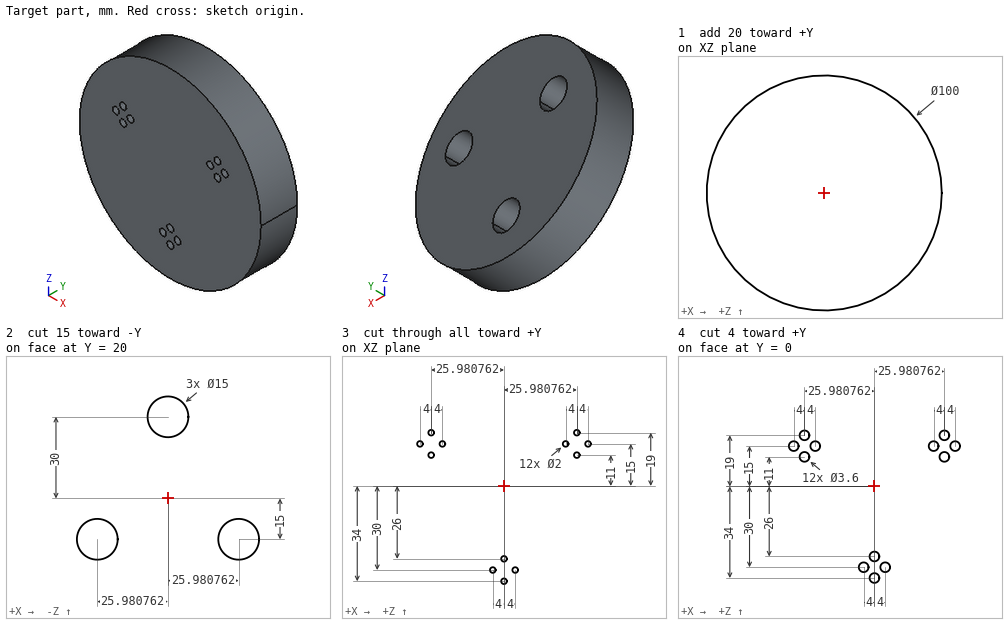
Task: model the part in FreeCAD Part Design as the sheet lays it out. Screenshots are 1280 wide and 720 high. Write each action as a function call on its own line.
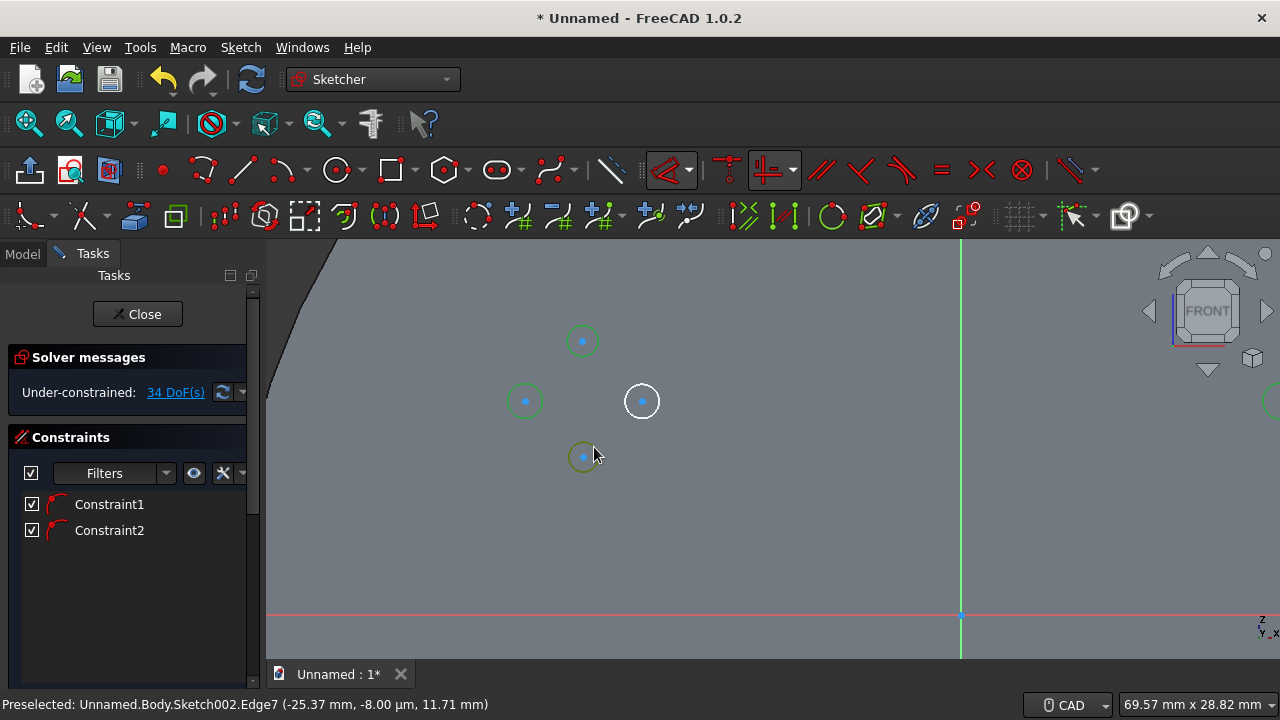
click(654, 389)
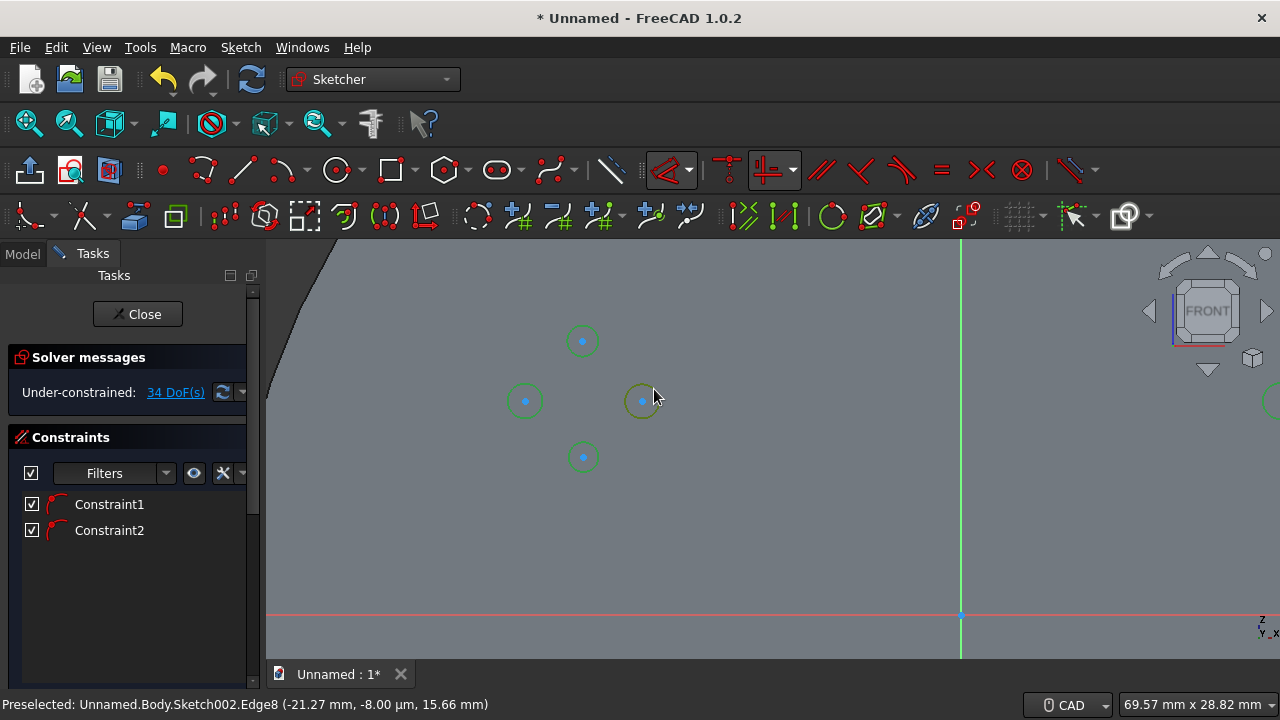
scroll(594, 330, down, 6)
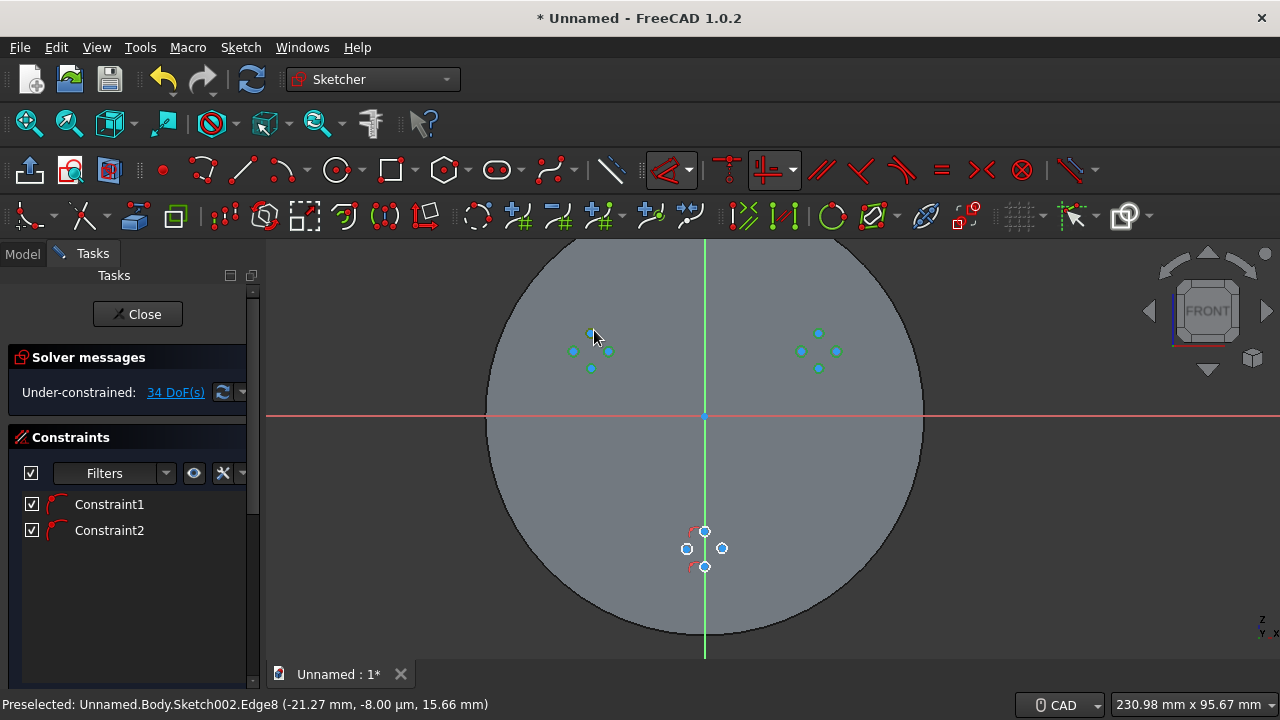
scroll(708, 528, up, 7)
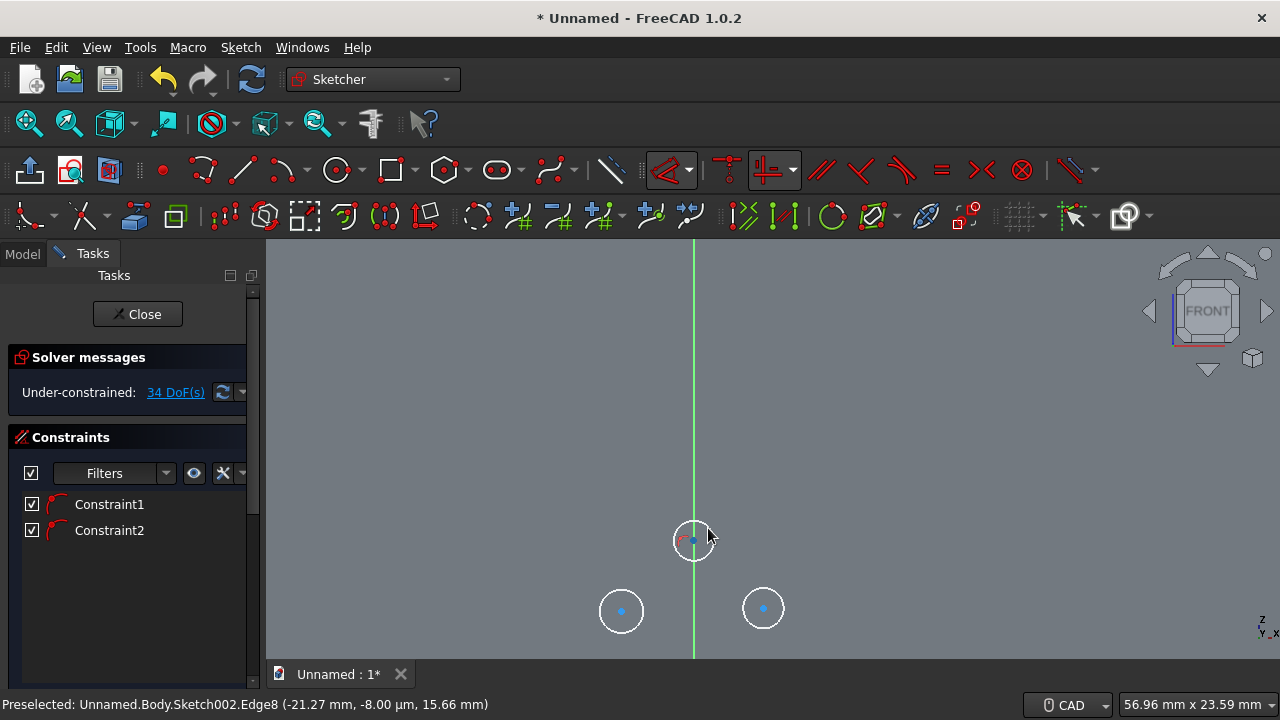
click(708, 527)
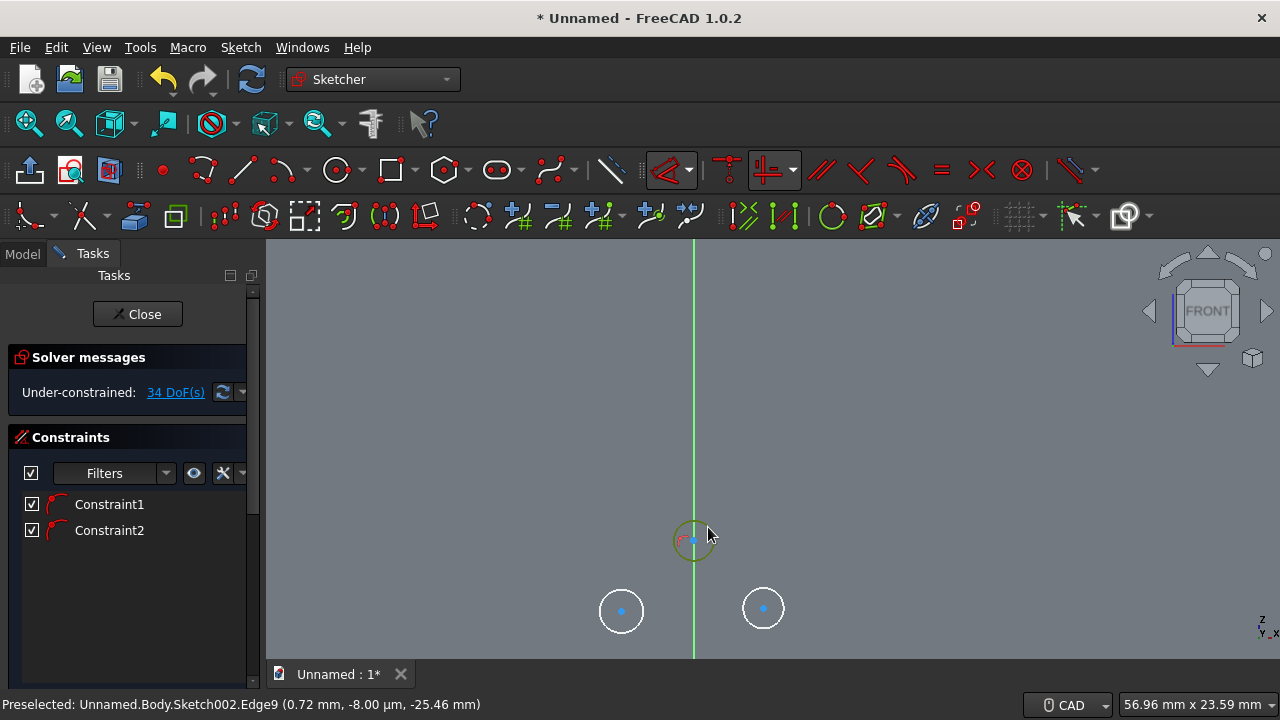
click(637, 596)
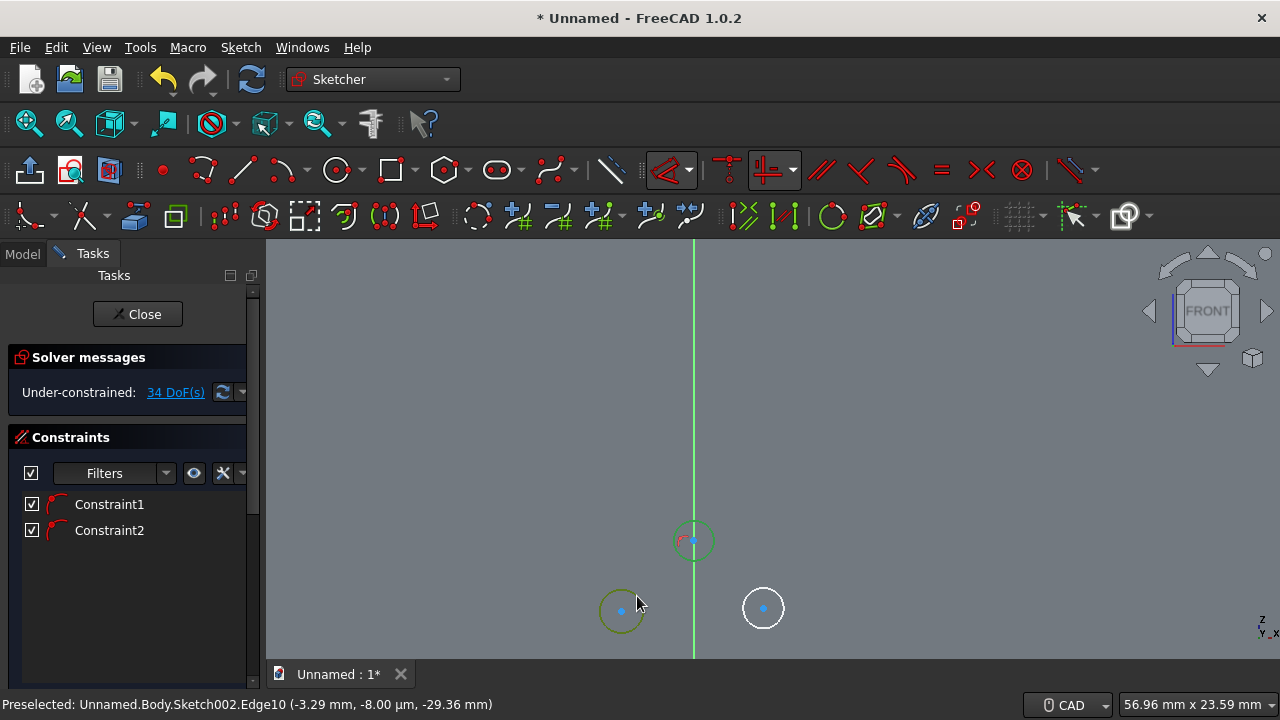
scroll(708, 529, down, 7)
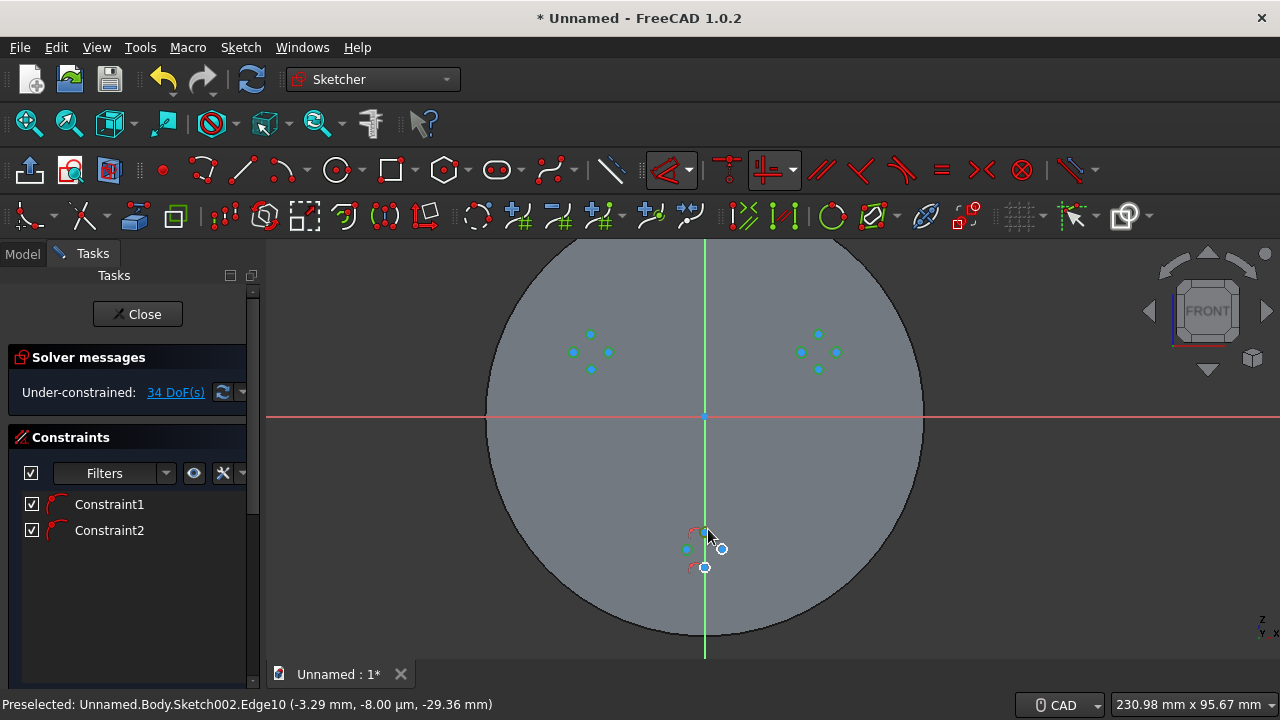
scroll(708, 564, up, 8)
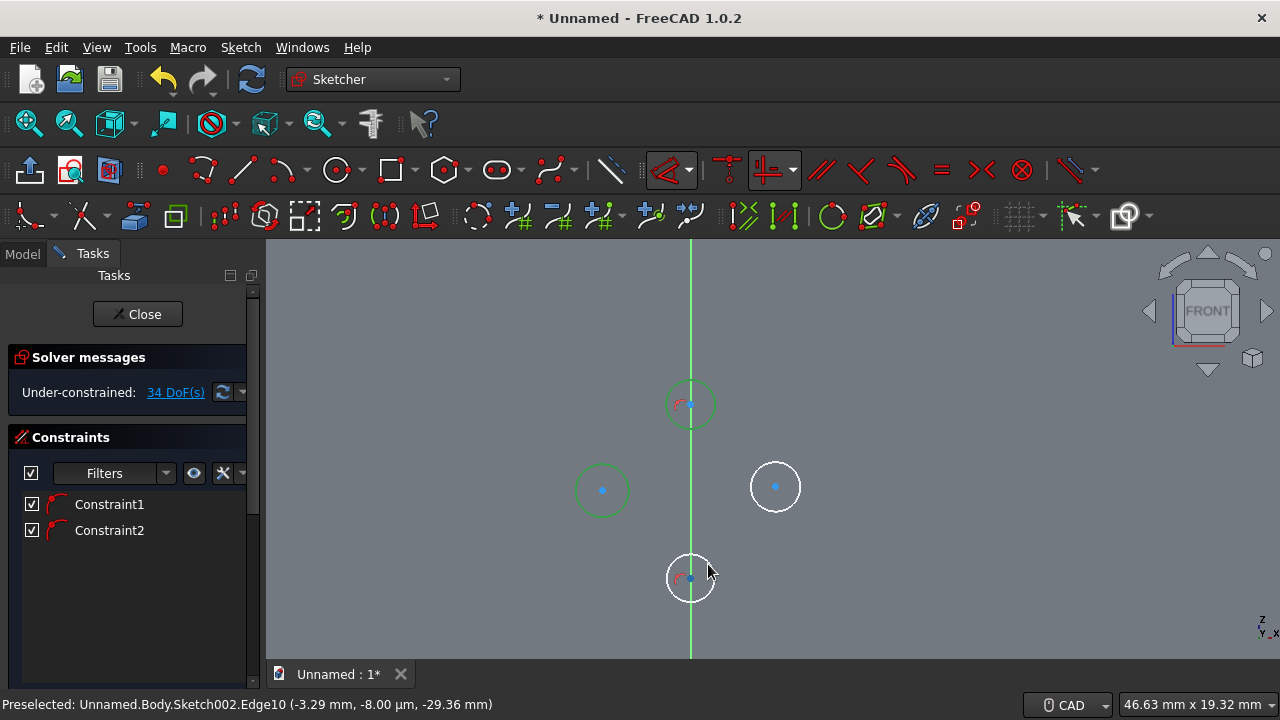
click(708, 561)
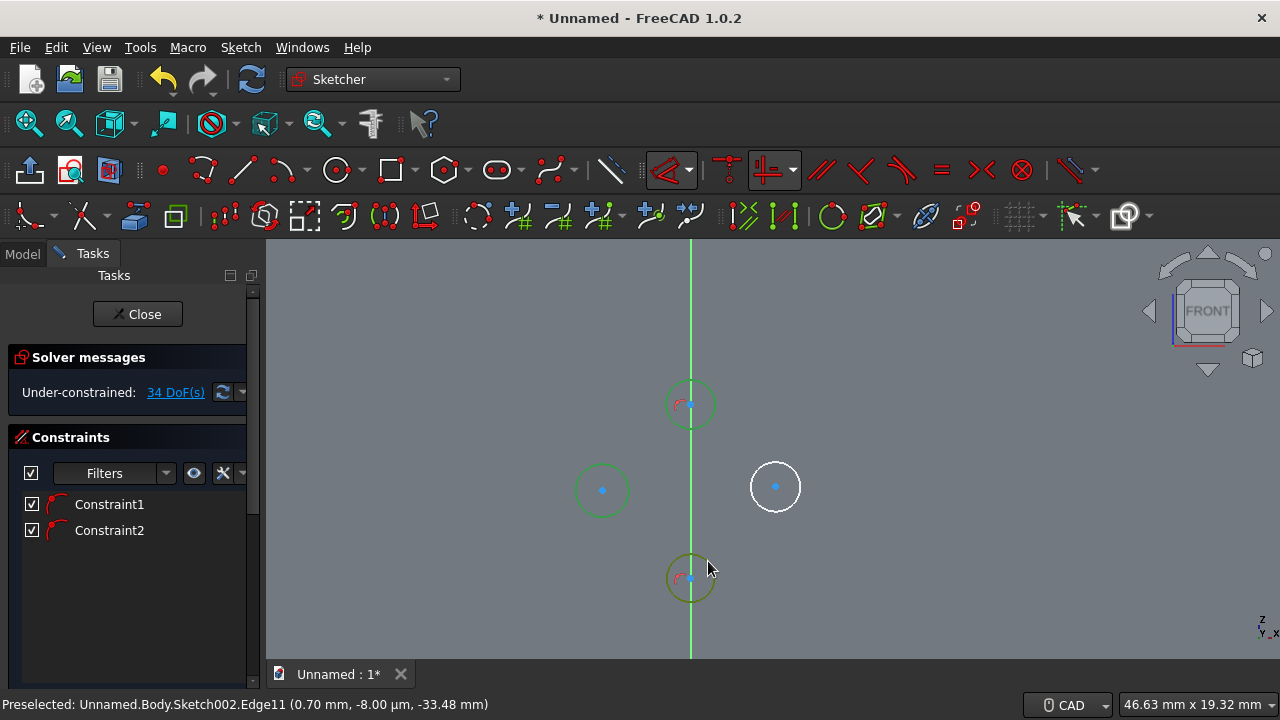
click(793, 469)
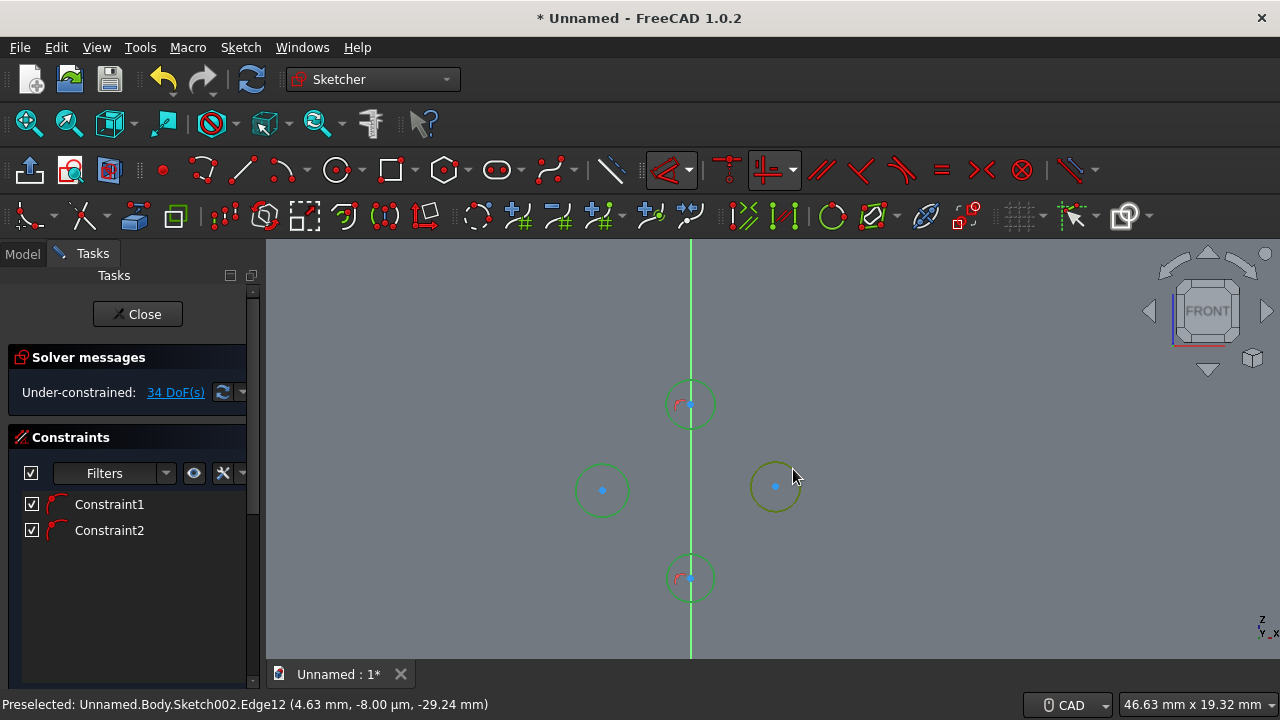
click(942, 170)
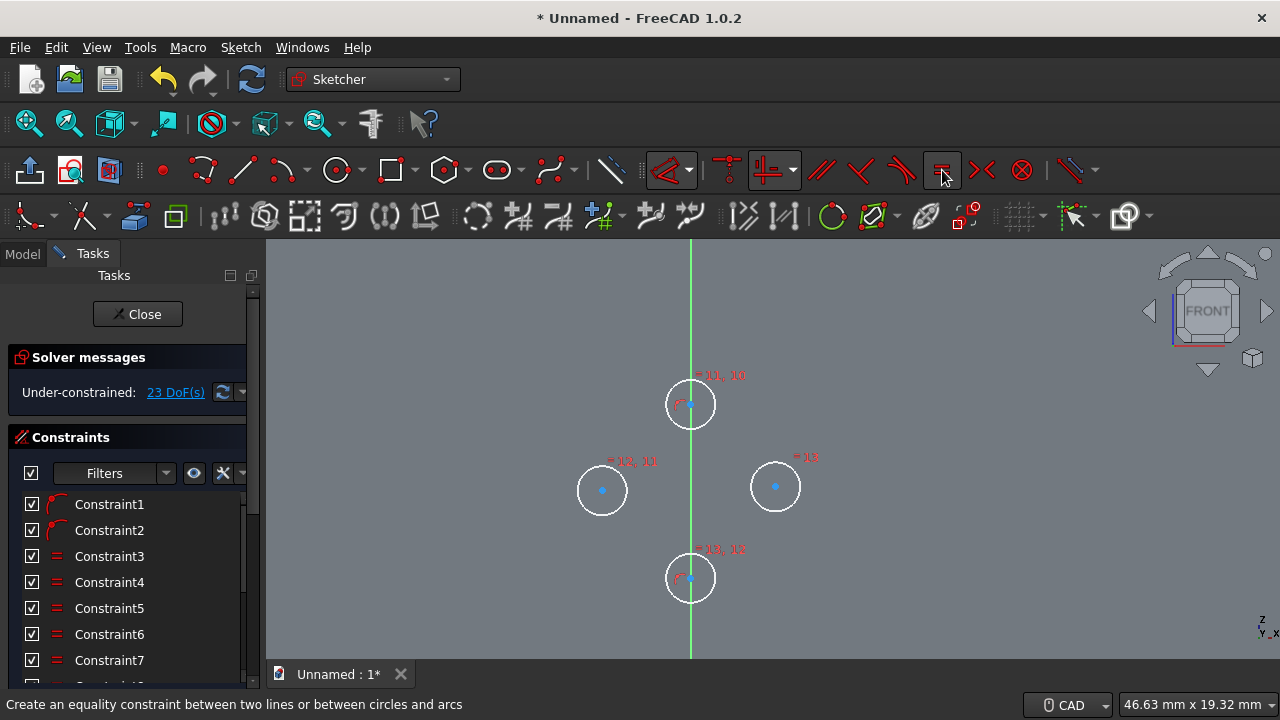
scroll(708, 564, down, 8)